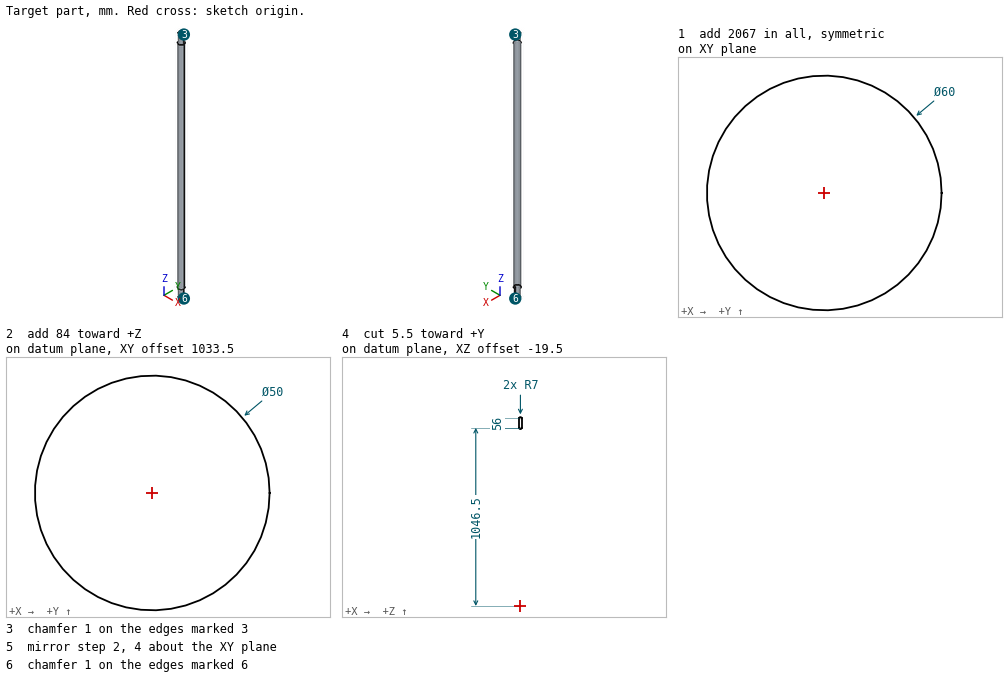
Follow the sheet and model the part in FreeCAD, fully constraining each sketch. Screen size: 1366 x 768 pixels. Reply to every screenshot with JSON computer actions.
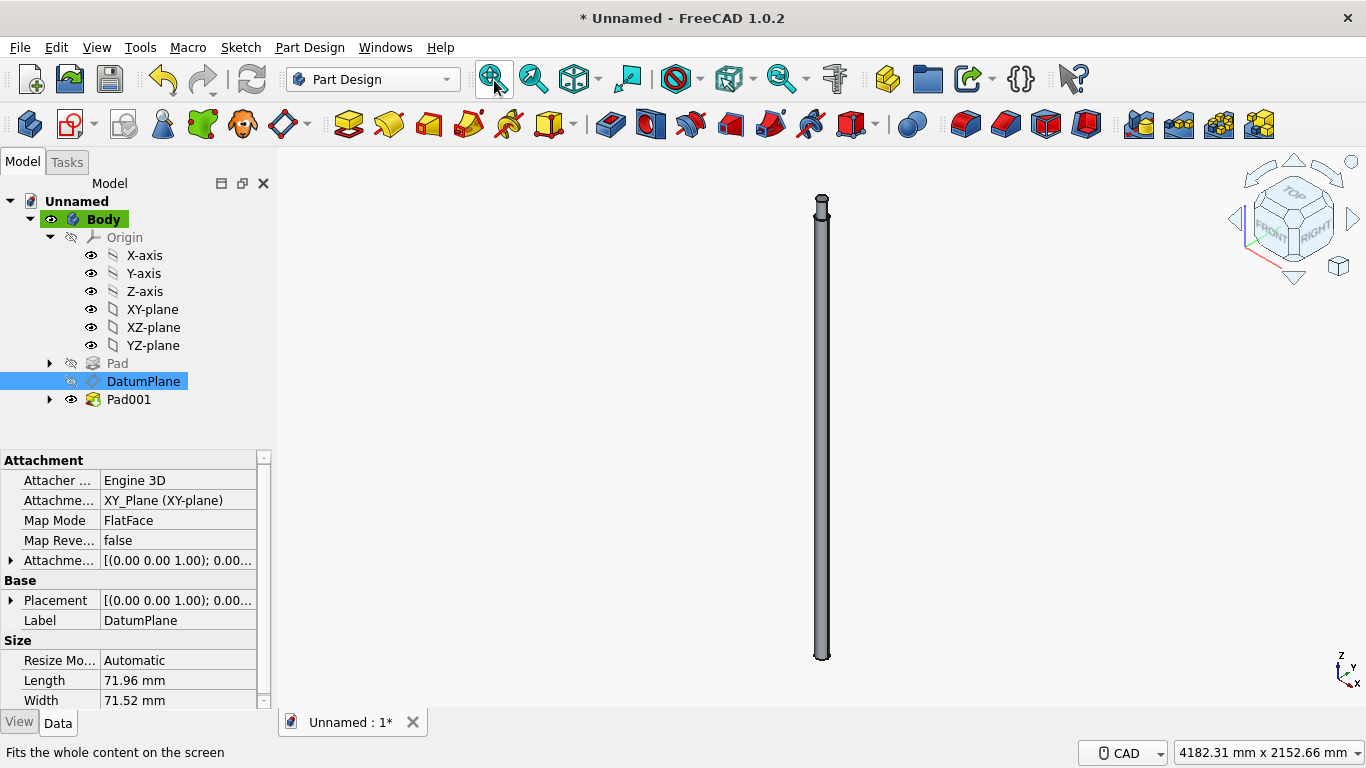
{"action": "left_click", "coordinate": [817, 195]}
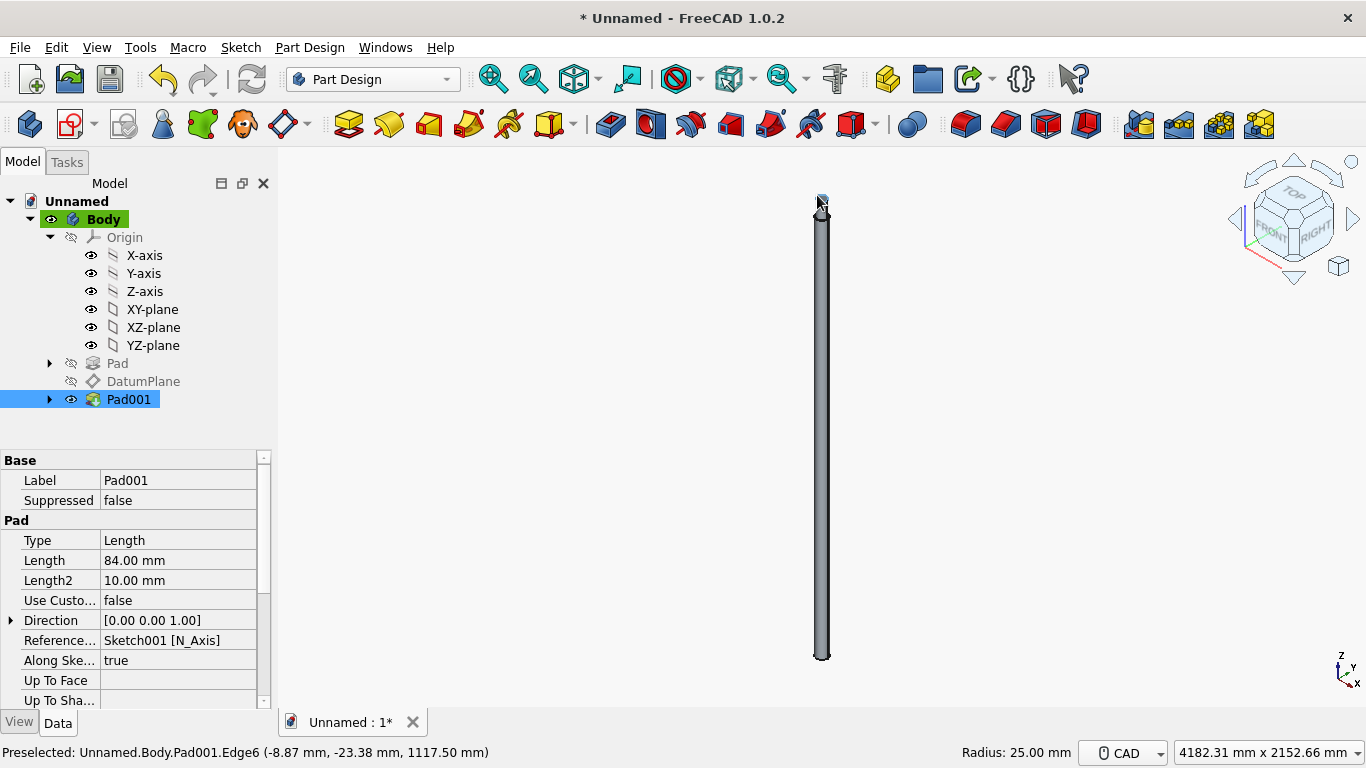
{"action": "left_click", "coordinate": [1006, 124]}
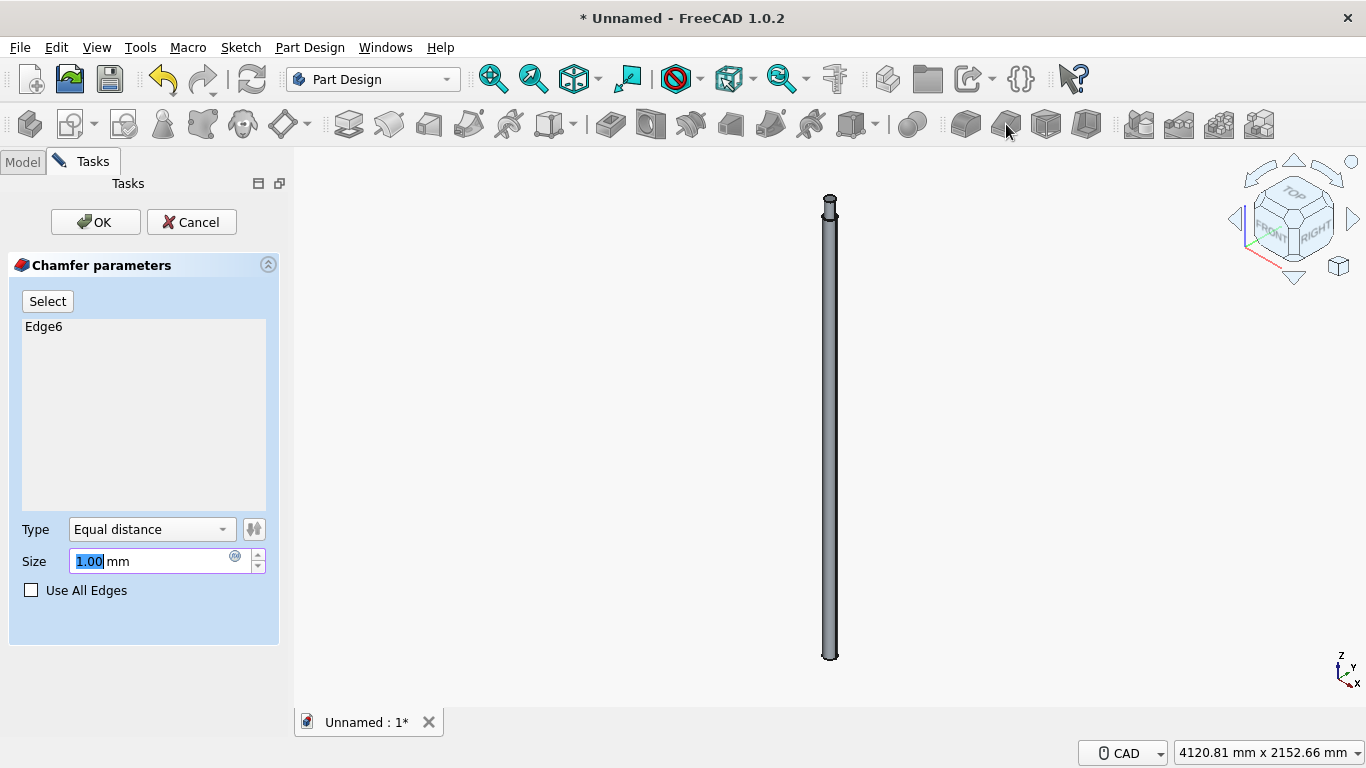
{"action": "type", "text": "1"}
{"action": "key", "text": "Tab"}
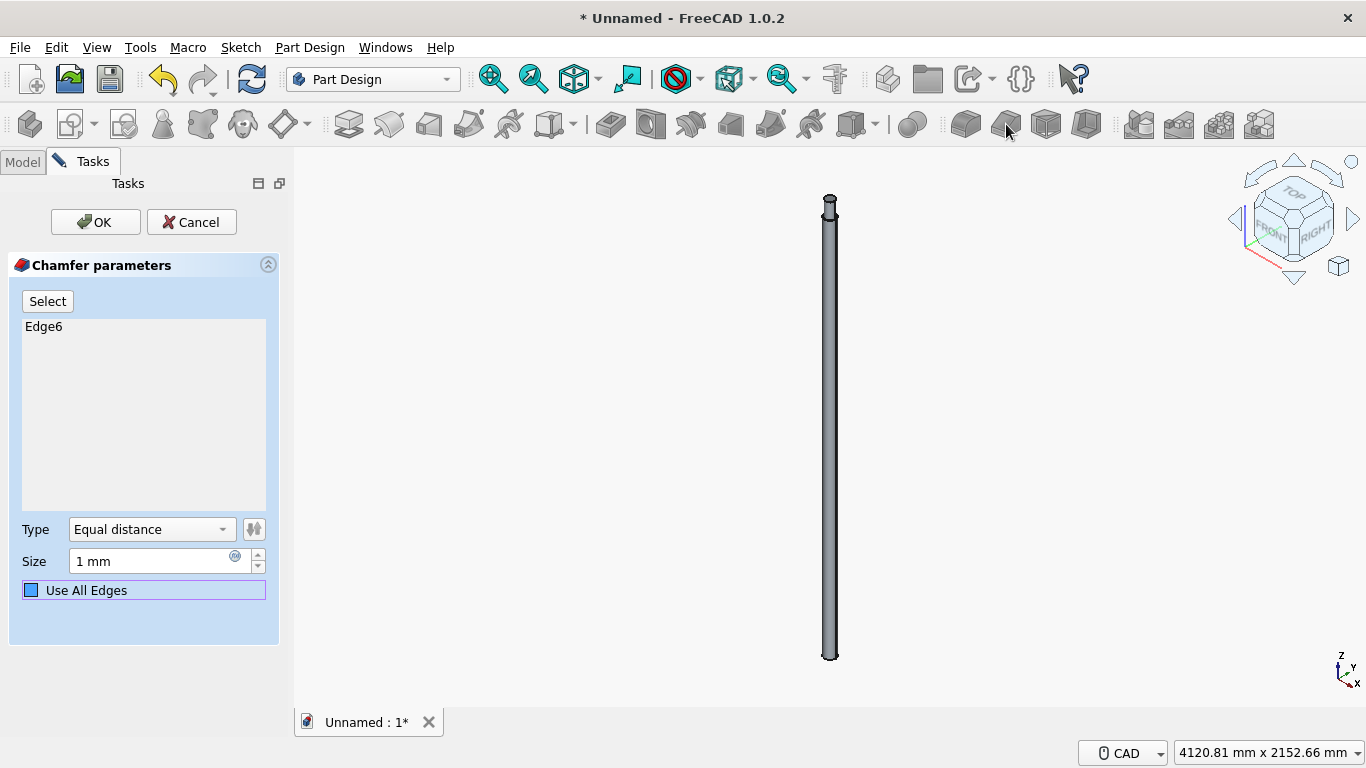
{"action": "left_click", "coordinate": [96, 222]}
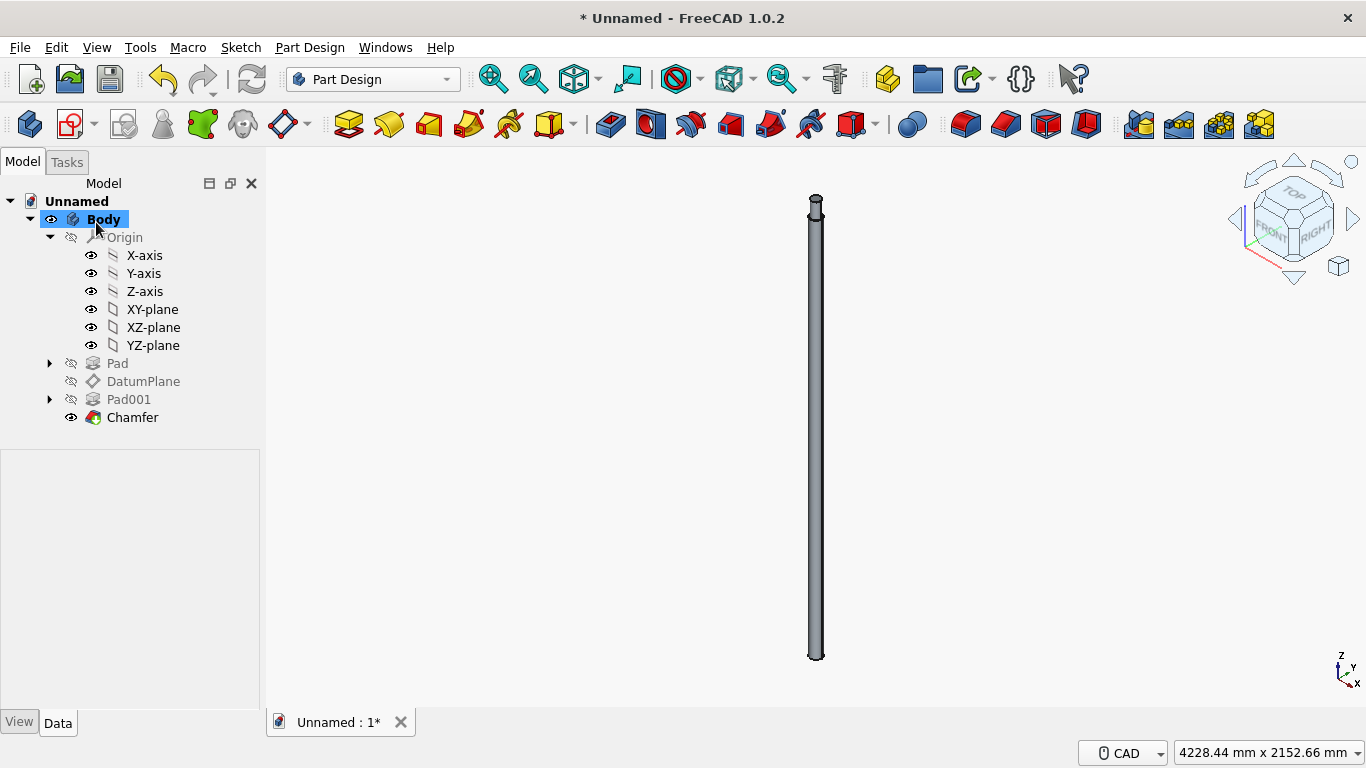
{"action": "left_click", "coordinate": [136, 327]}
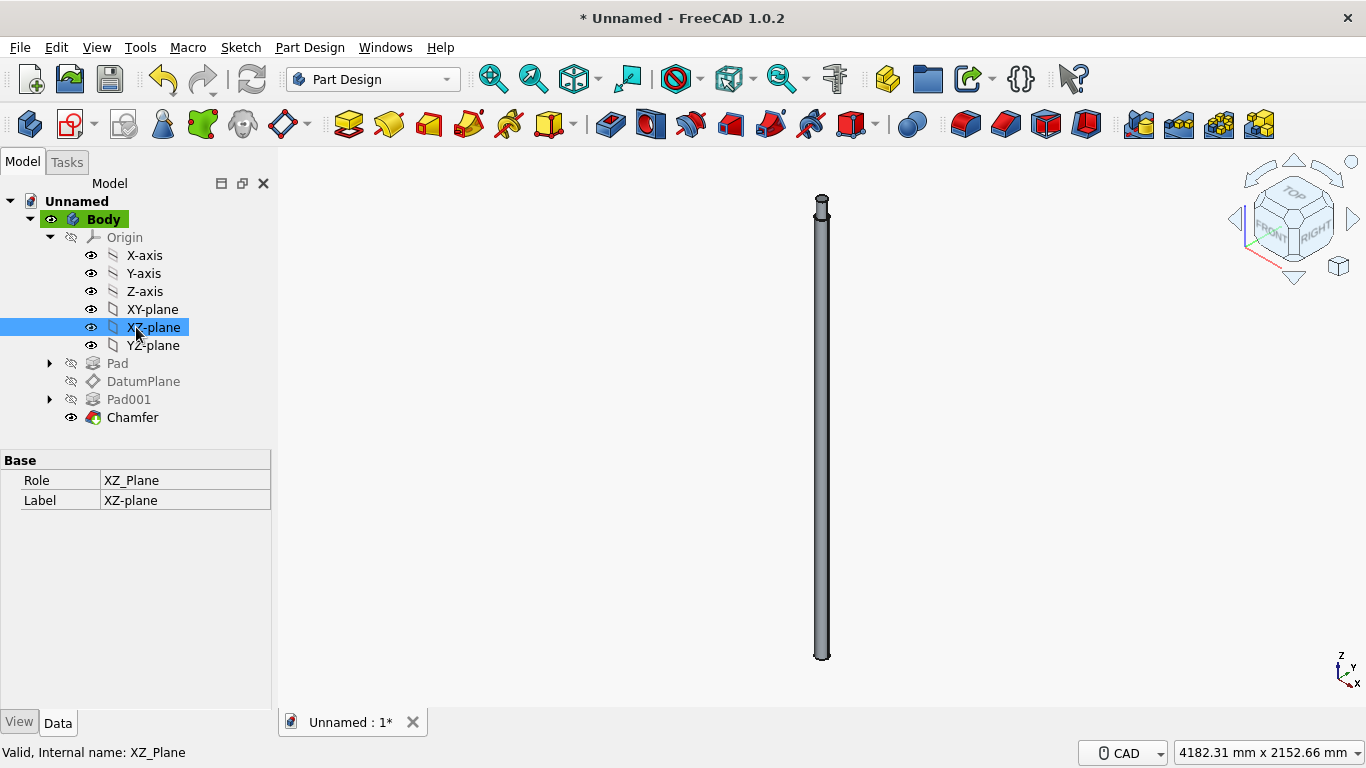
{"action": "left_click", "coordinate": [284, 124]}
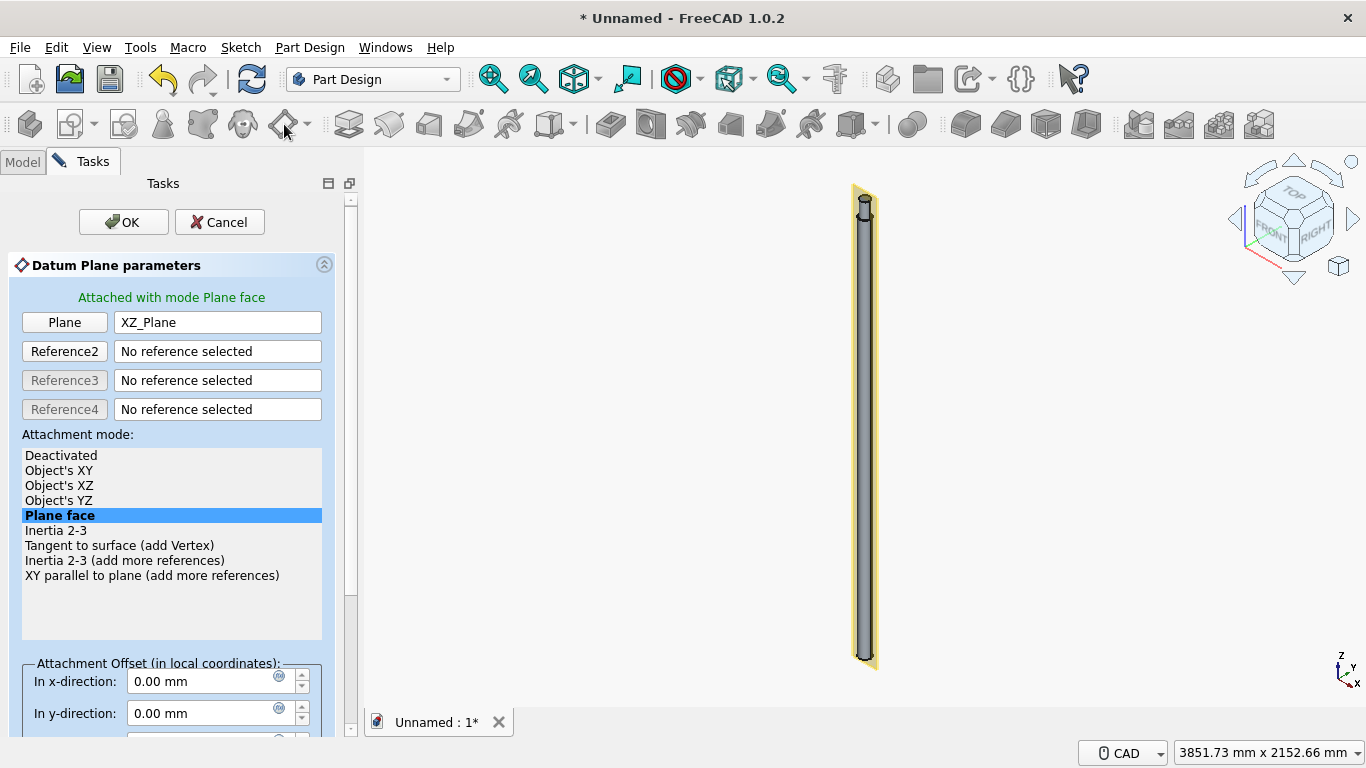
{"action": "scroll", "coordinate": [351, 464], "scroll_direction": "down", "scroll_amount": 2}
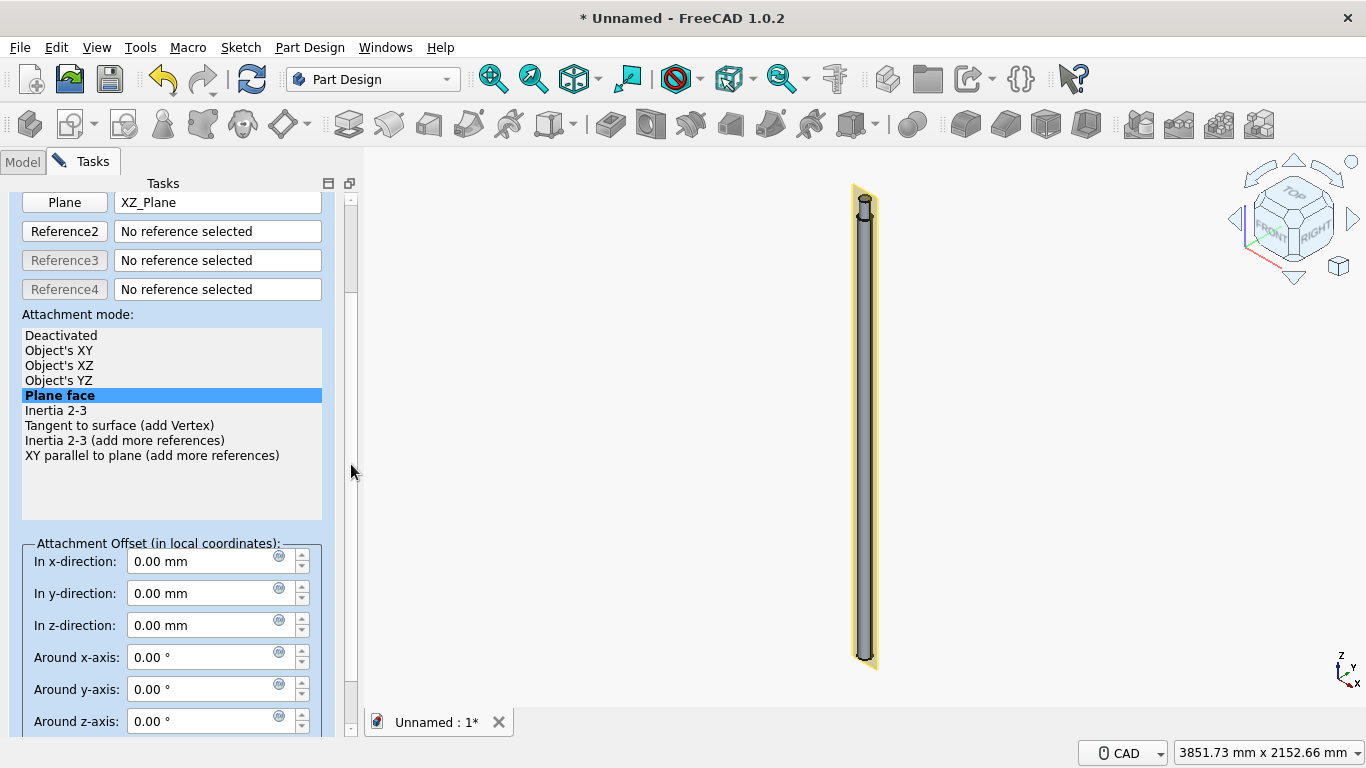
{"action": "triple_click", "coordinate": [210, 625]}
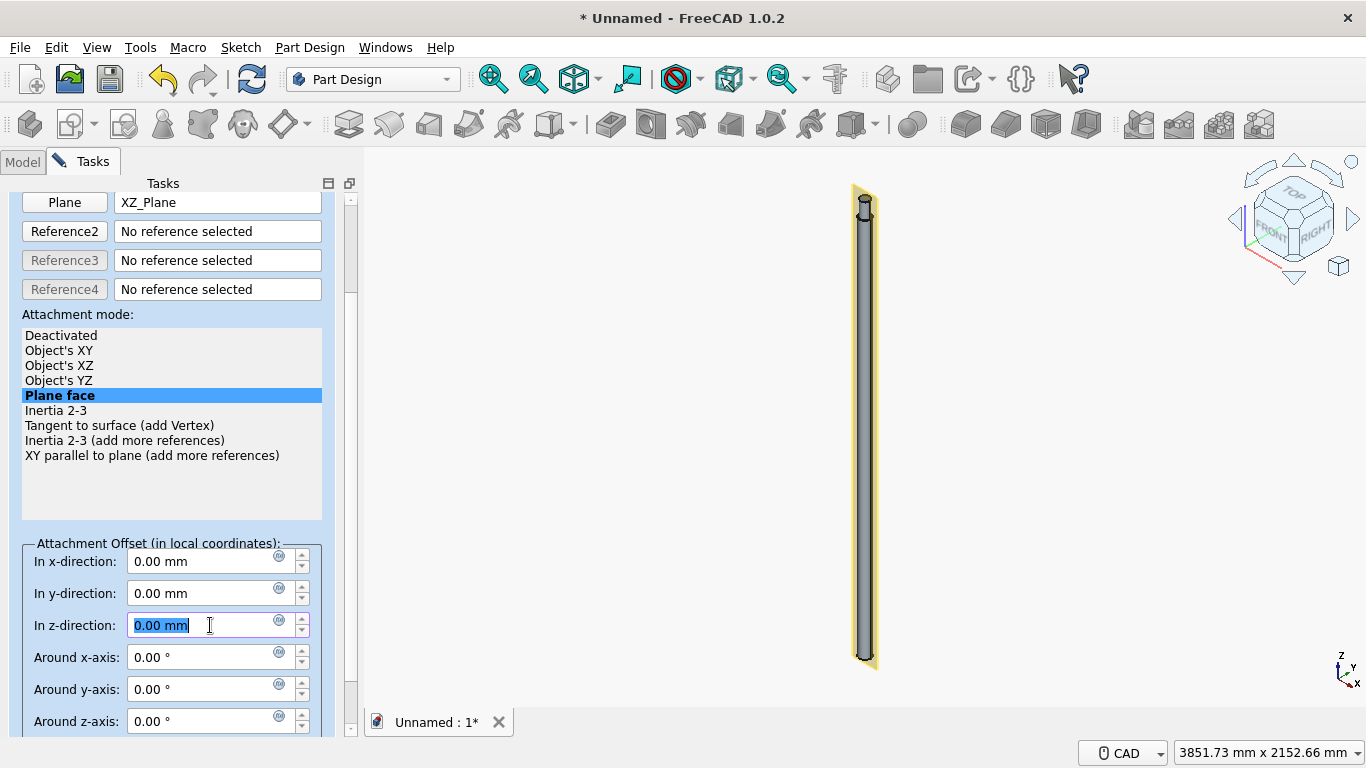
{"action": "type", "text": "-19.5"}
{"action": "key", "text": "Tab"}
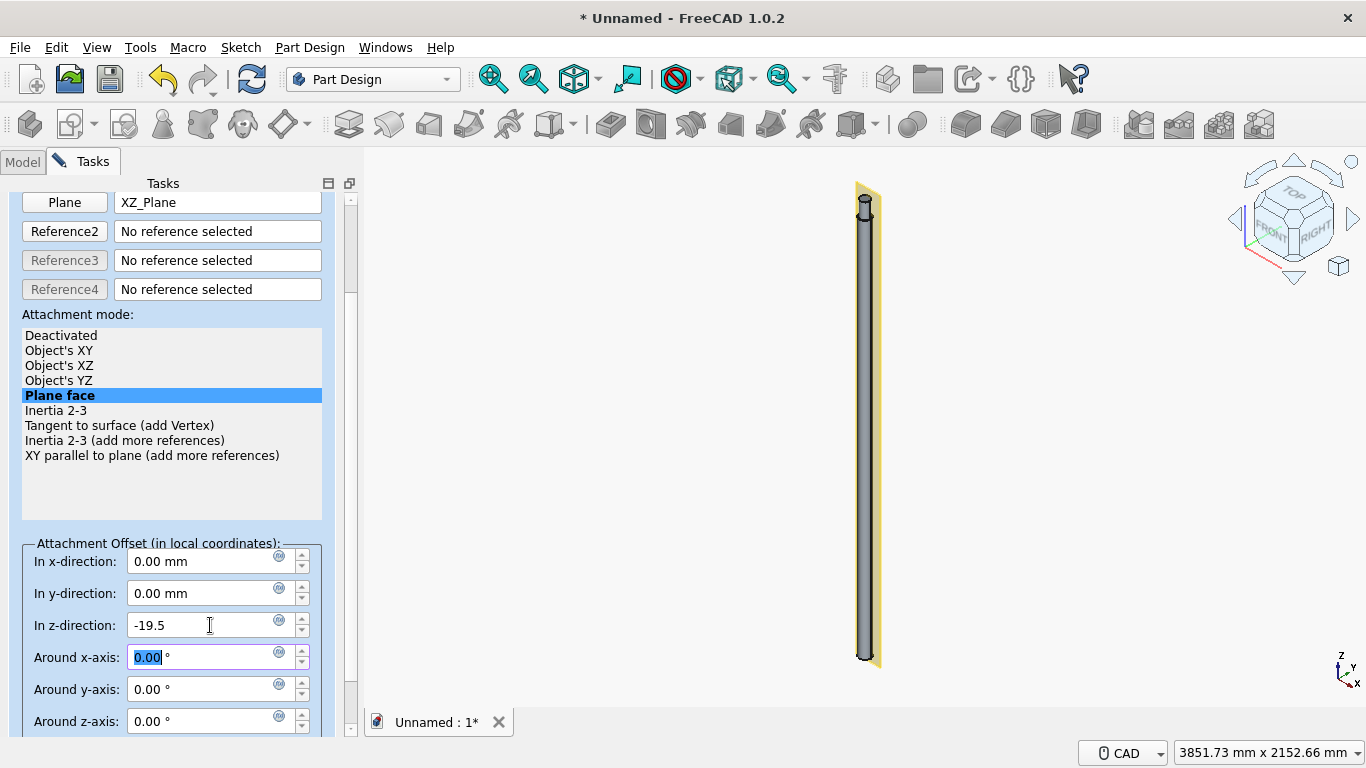
{"action": "scroll", "coordinate": [351, 464], "scroll_direction": "up", "scroll_amount": 3}